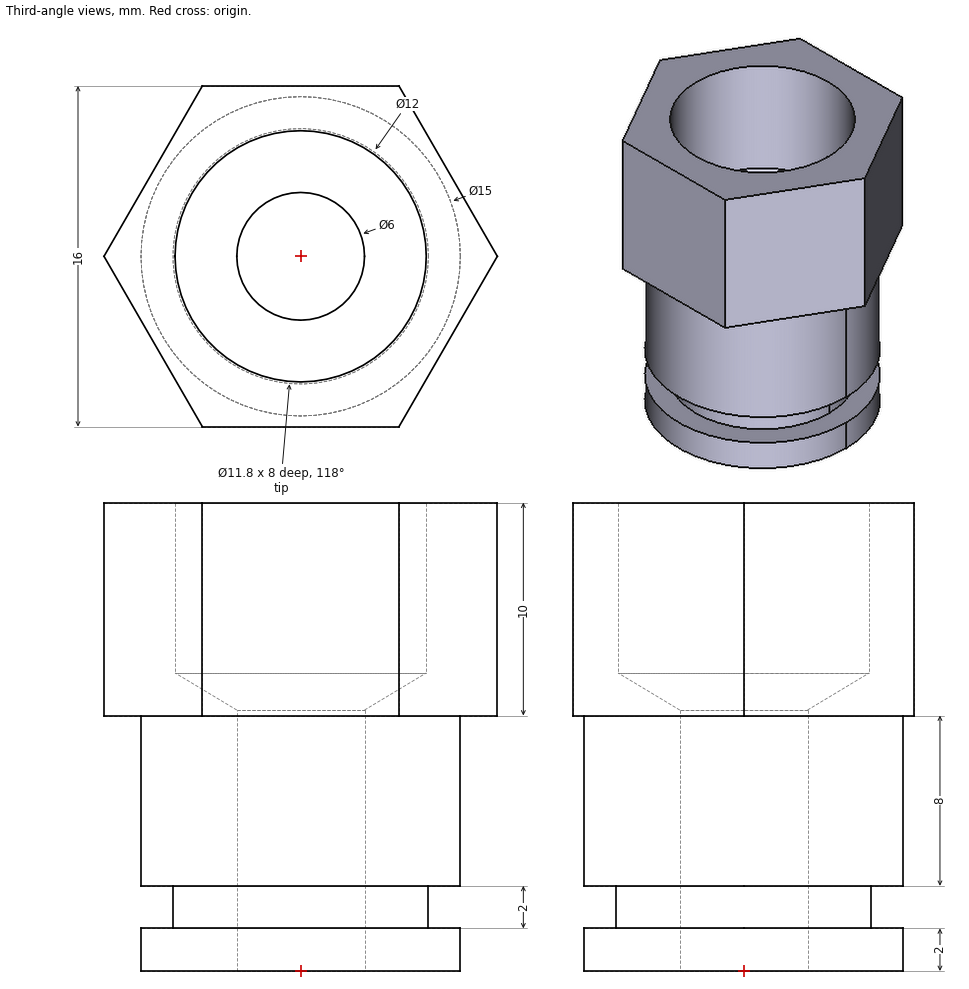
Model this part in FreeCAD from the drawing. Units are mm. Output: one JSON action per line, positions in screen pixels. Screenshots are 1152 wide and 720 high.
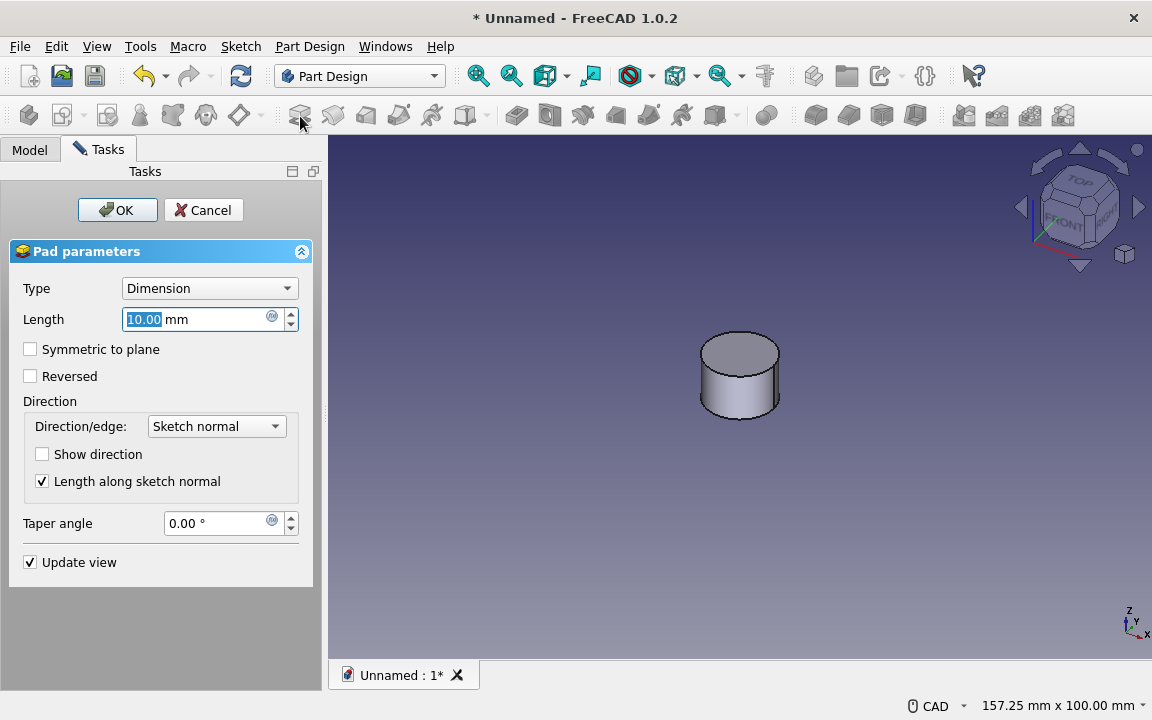
{"action": "type", "text": "2"}
{"action": "key", "text": "Tab"}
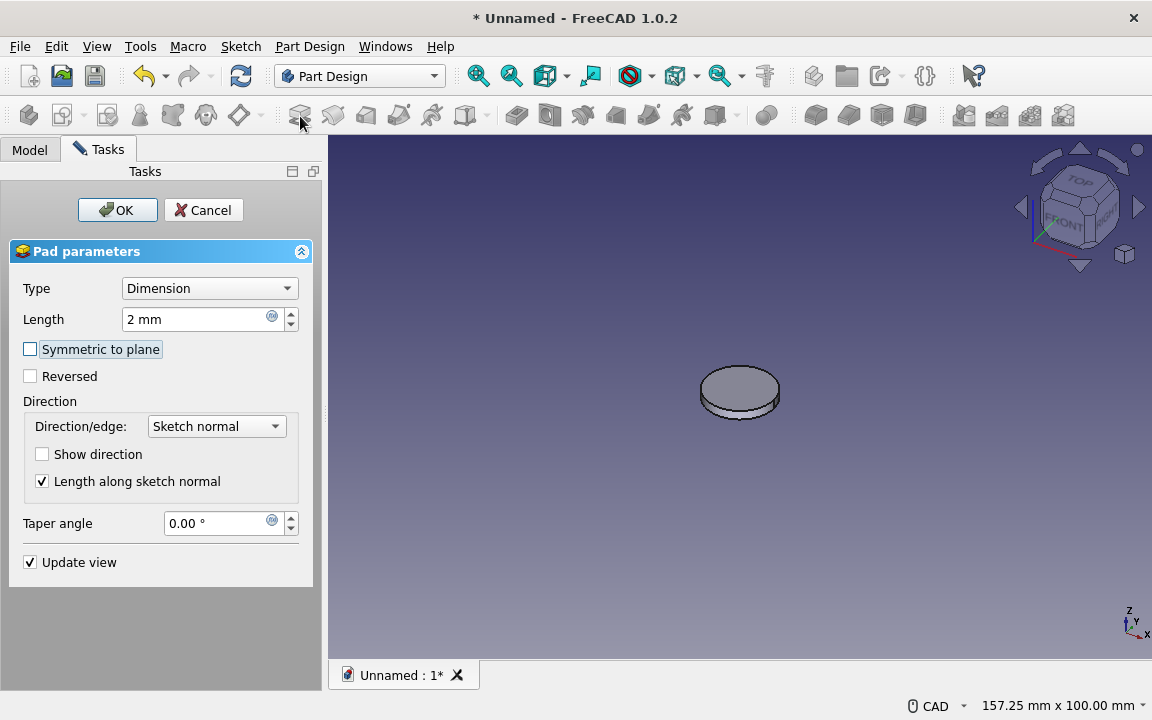
{"action": "left_click", "coordinate": [118, 210]}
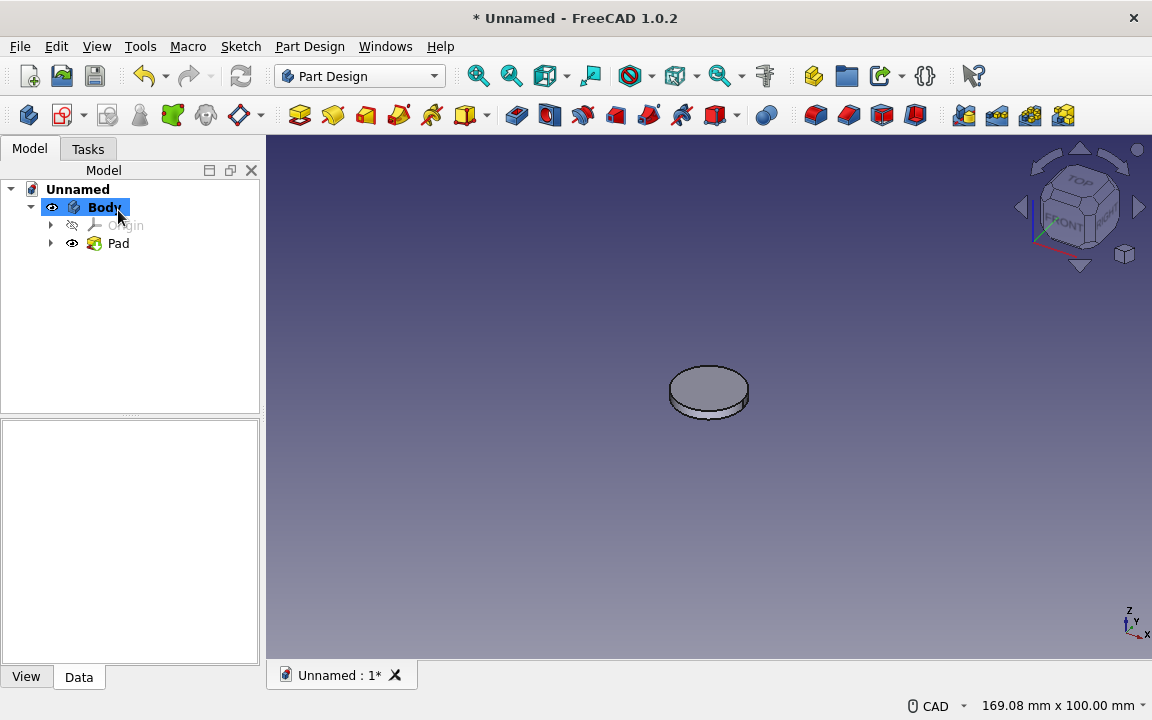
{"action": "left_click", "coordinate": [479, 76]}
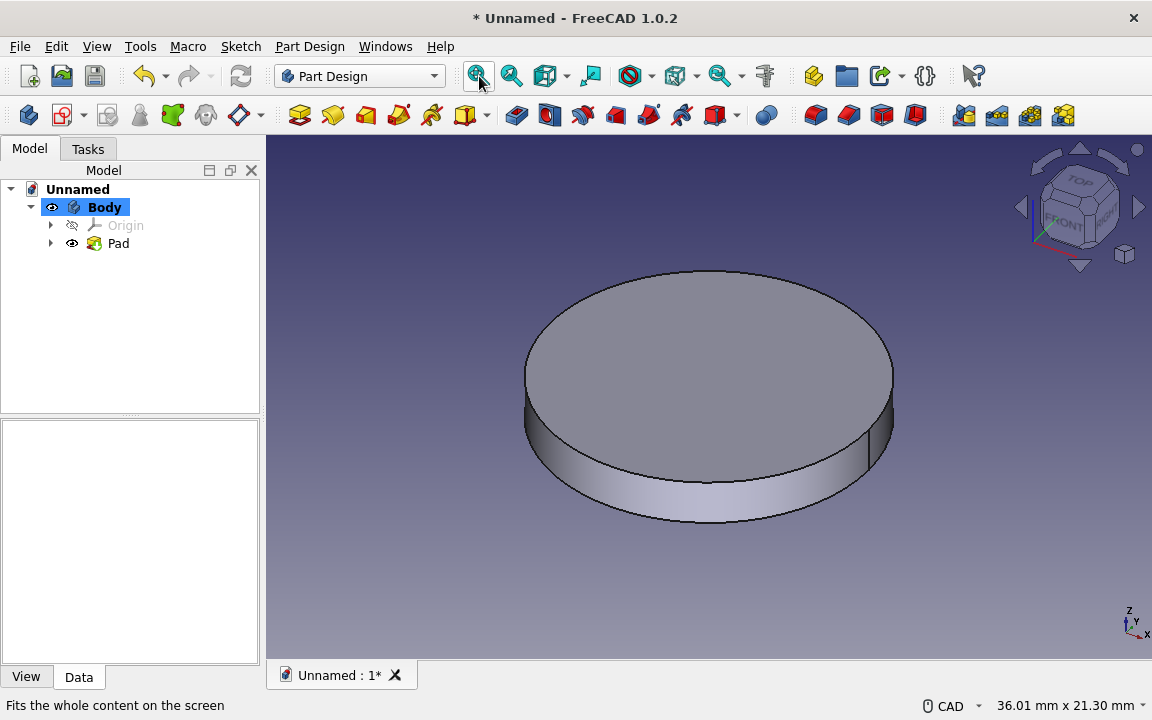
{"action": "left_click", "coordinate": [709, 376]}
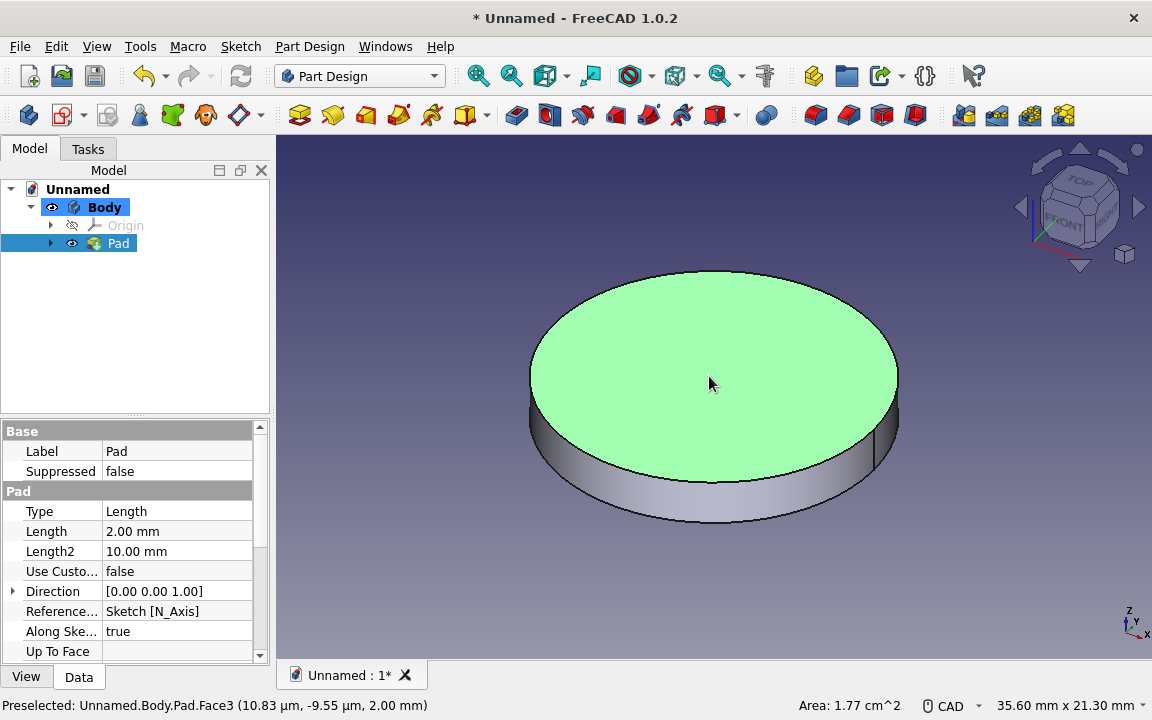
{"action": "left_click", "coordinate": [62, 116]}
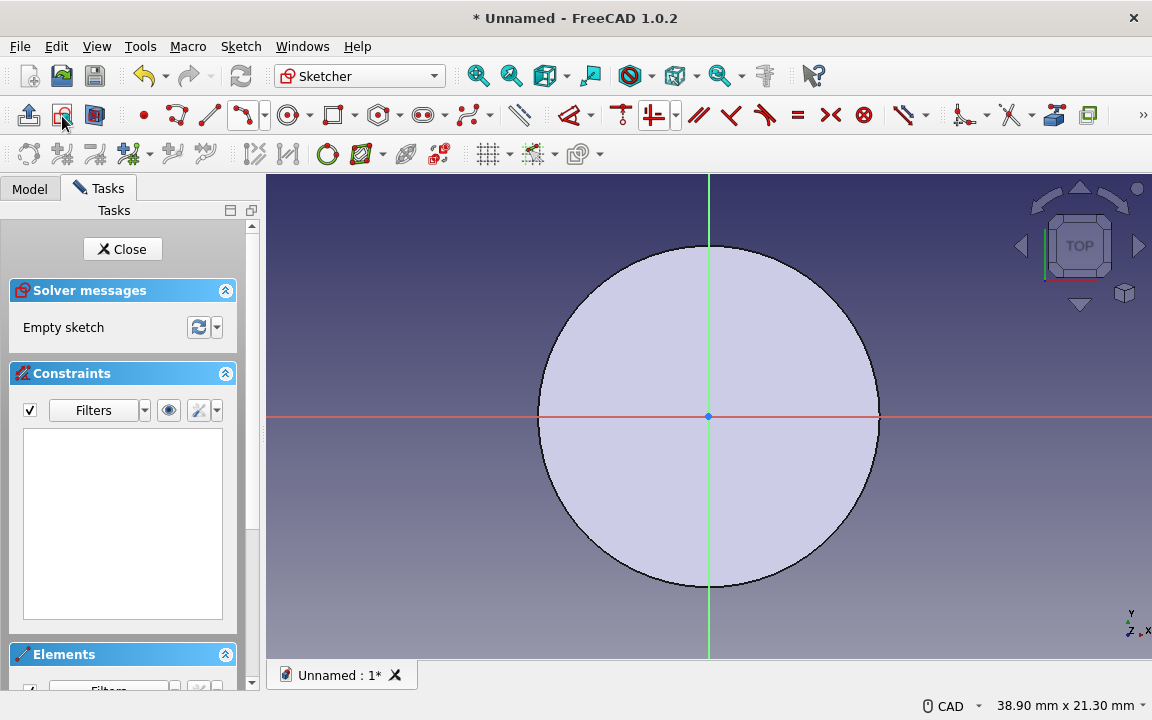
{"action": "left_click", "coordinate": [288, 116]}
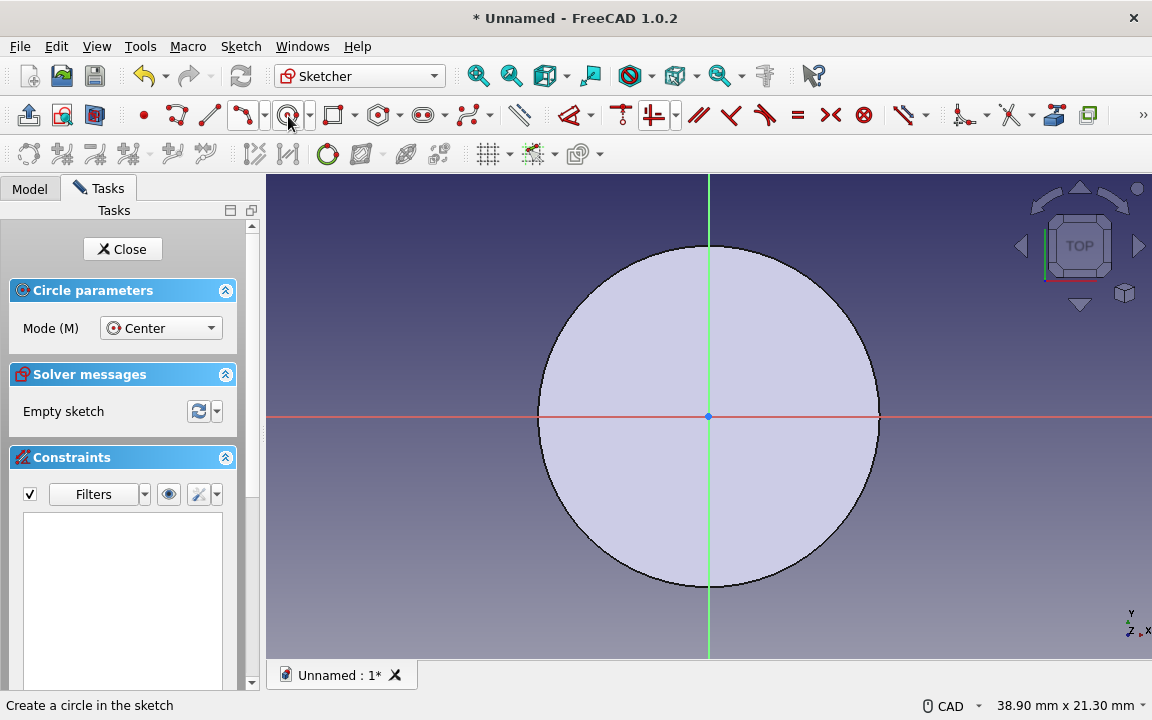
{"action": "left_click", "coordinate": [709, 416]}
{"action": "left_click", "coordinate": [806, 320]}
{"action": "key", "text": "Escape"}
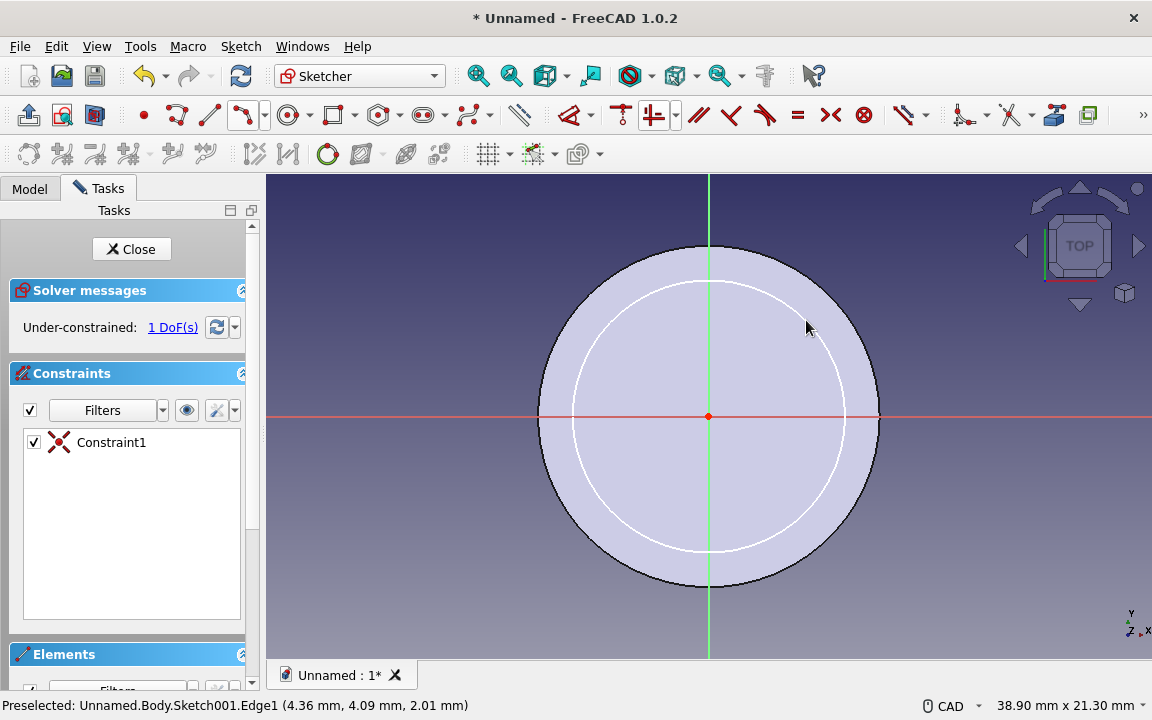
{"action": "left_click", "coordinate": [568, 116]}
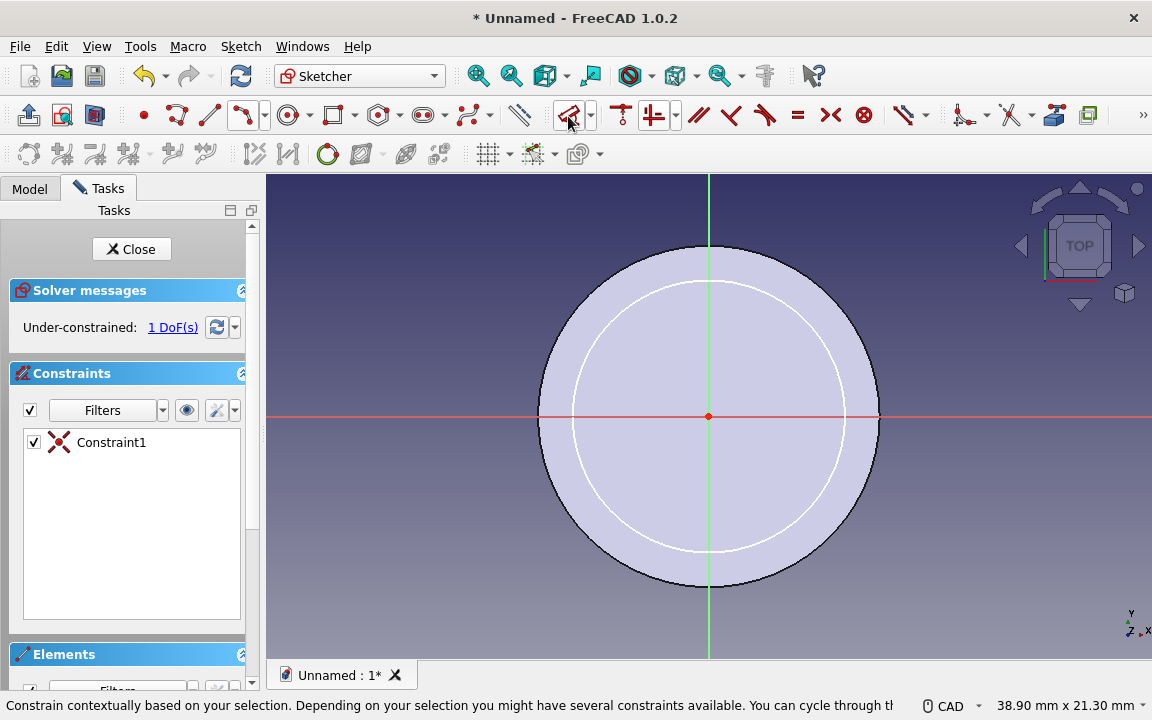
{"action": "left_click", "coordinate": [805, 320]}
{"action": "left_click", "coordinate": [828, 297]}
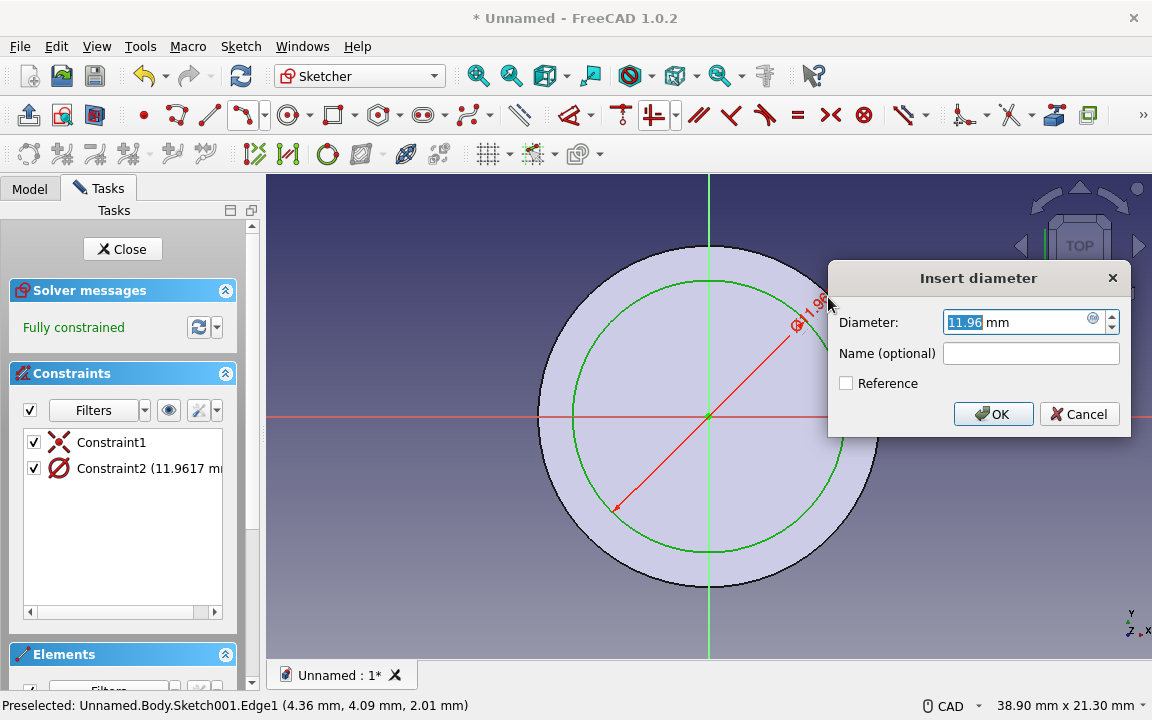
{"action": "type", "text": "12"}
{"action": "key", "text": "Return"}
{"action": "key", "text": "Escape"}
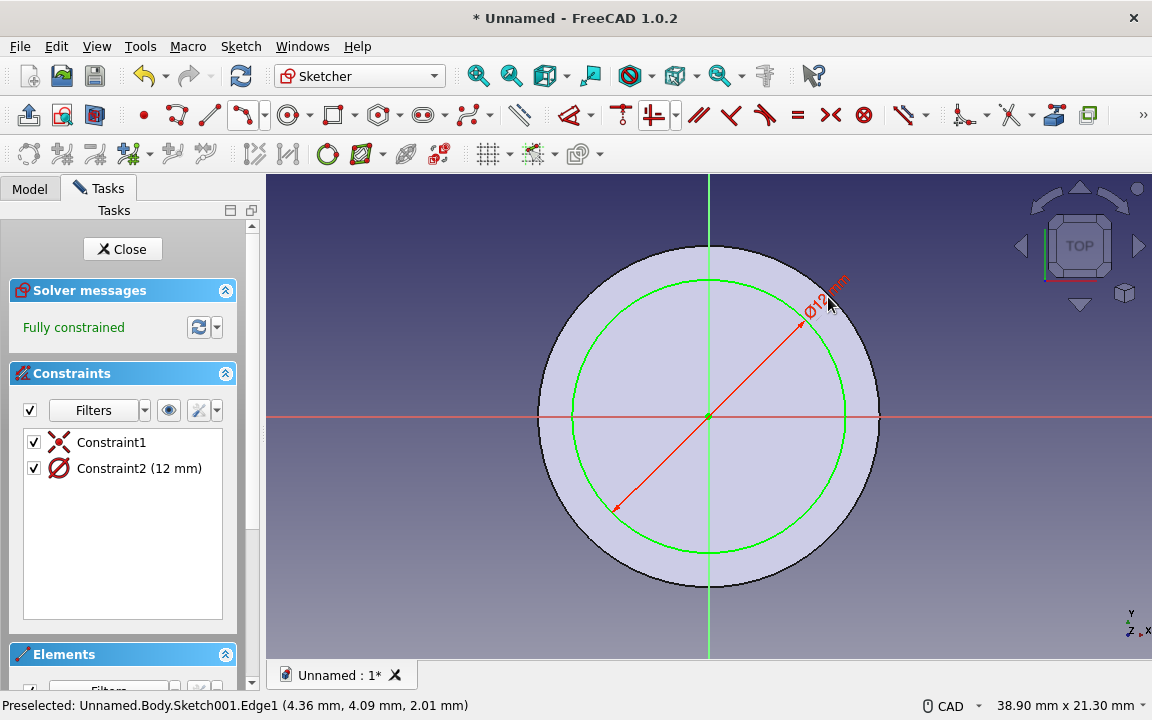
{"action": "left_click", "coordinate": [123, 249]}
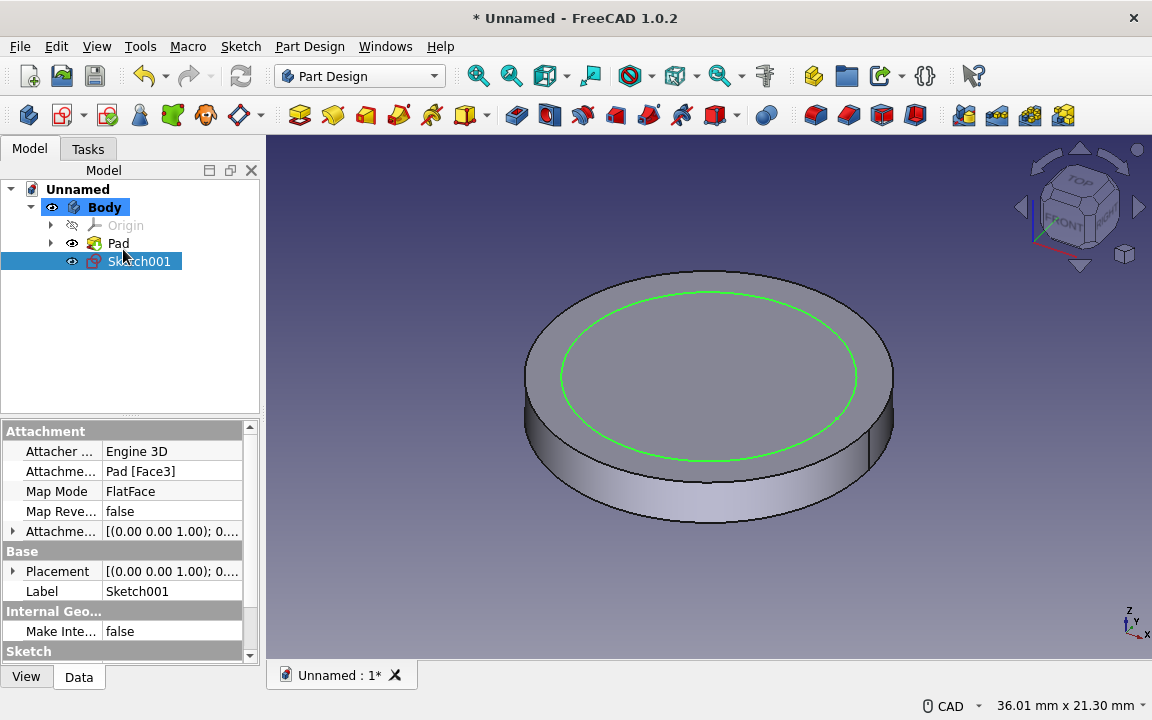
{"action": "left_click", "coordinate": [300, 116]}